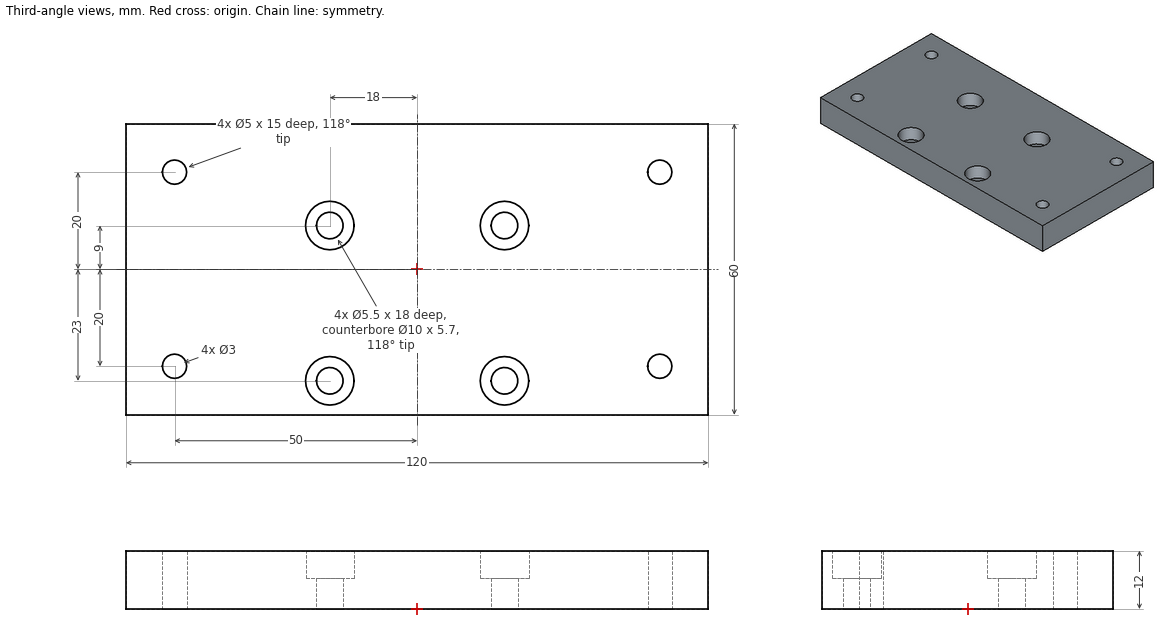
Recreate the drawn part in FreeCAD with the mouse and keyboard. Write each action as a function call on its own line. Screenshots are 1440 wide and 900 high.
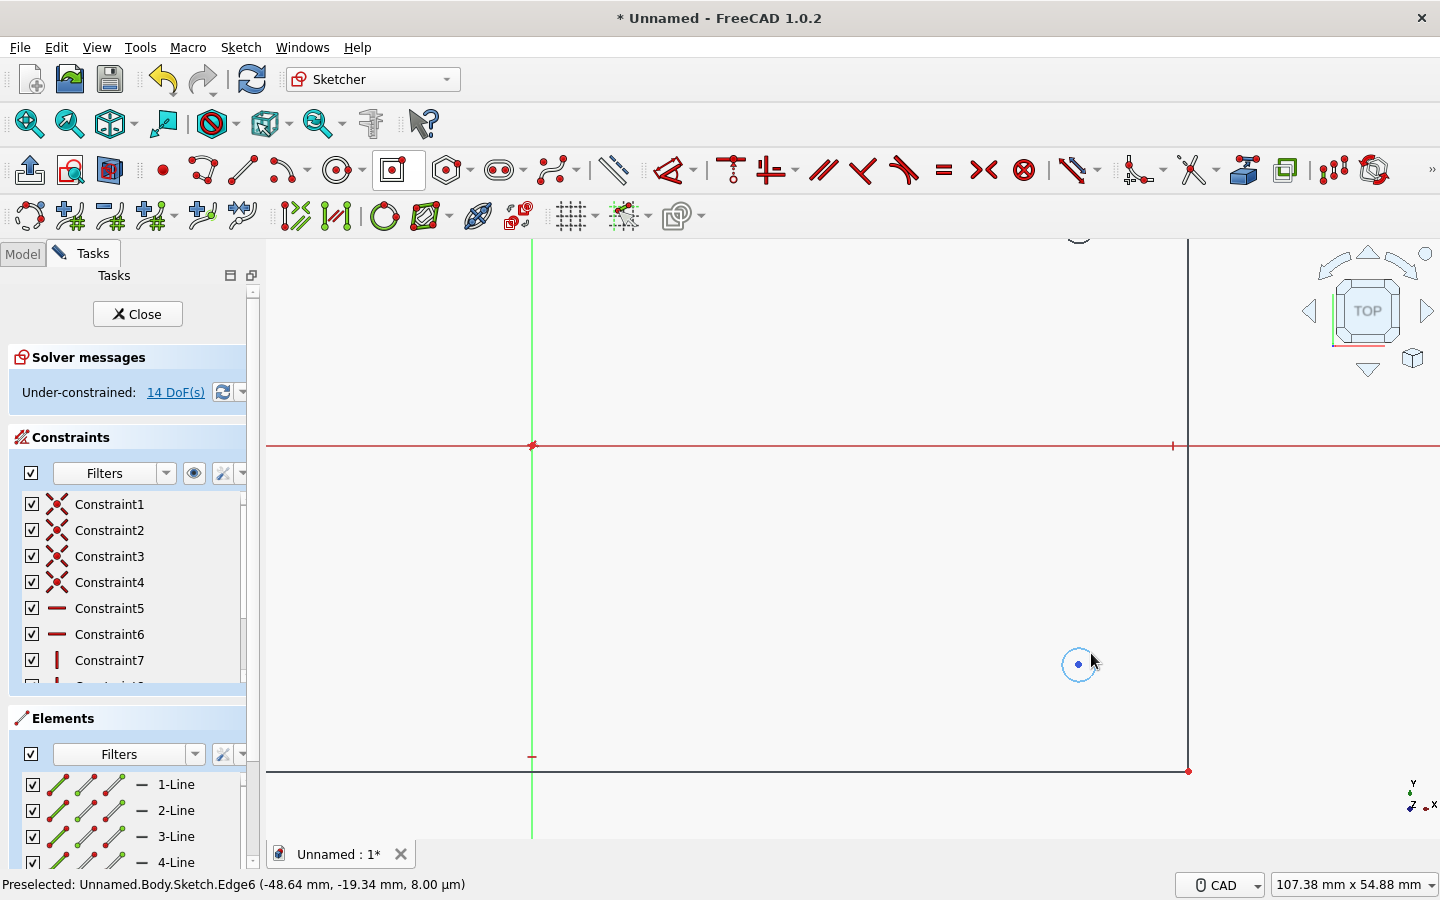
click(1091, 653)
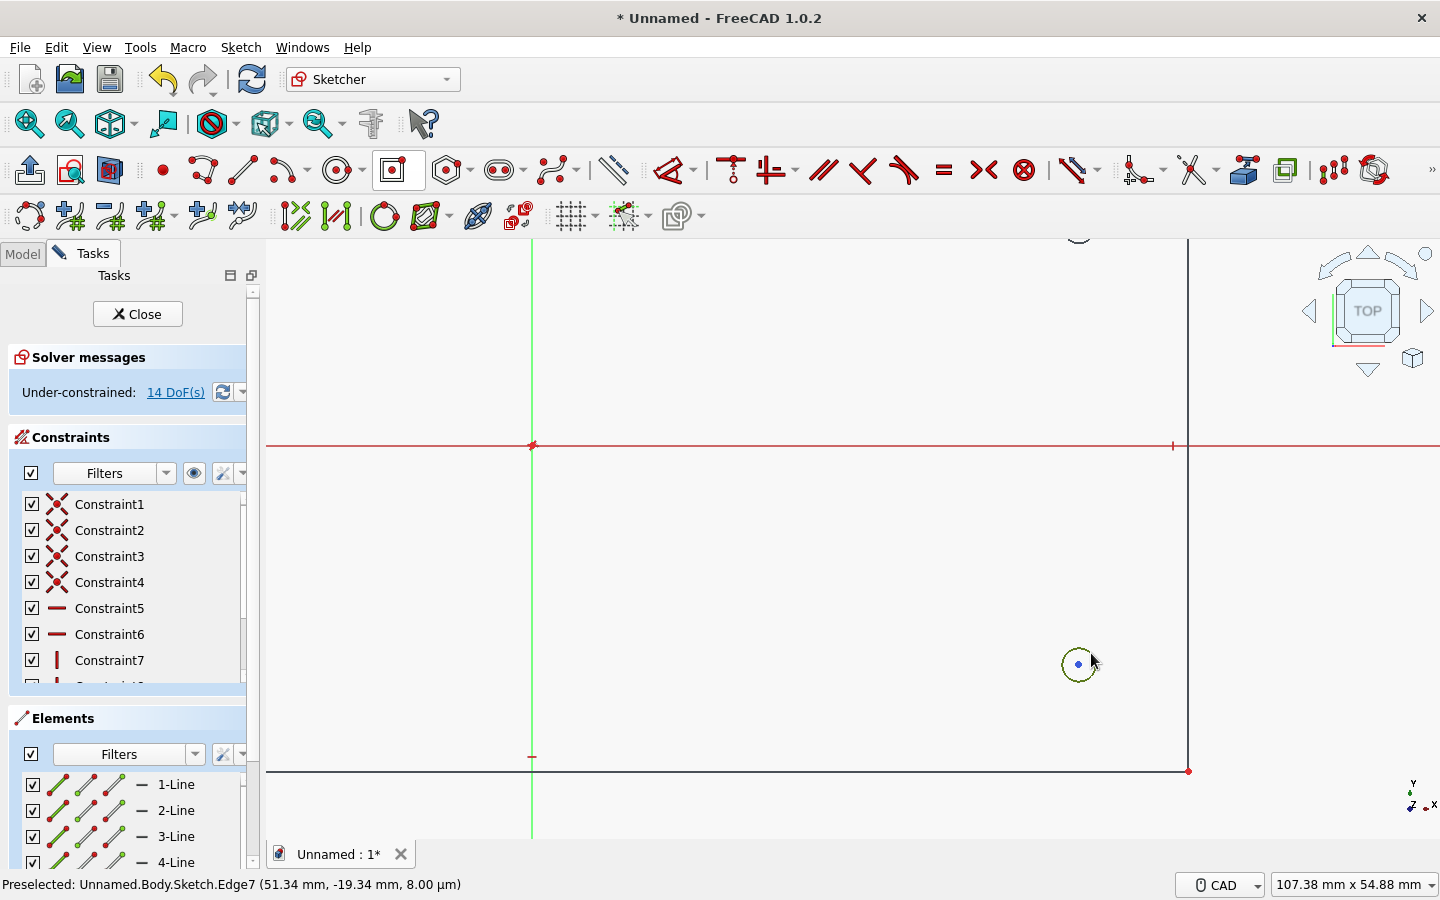
scroll(1091, 653, down, 3)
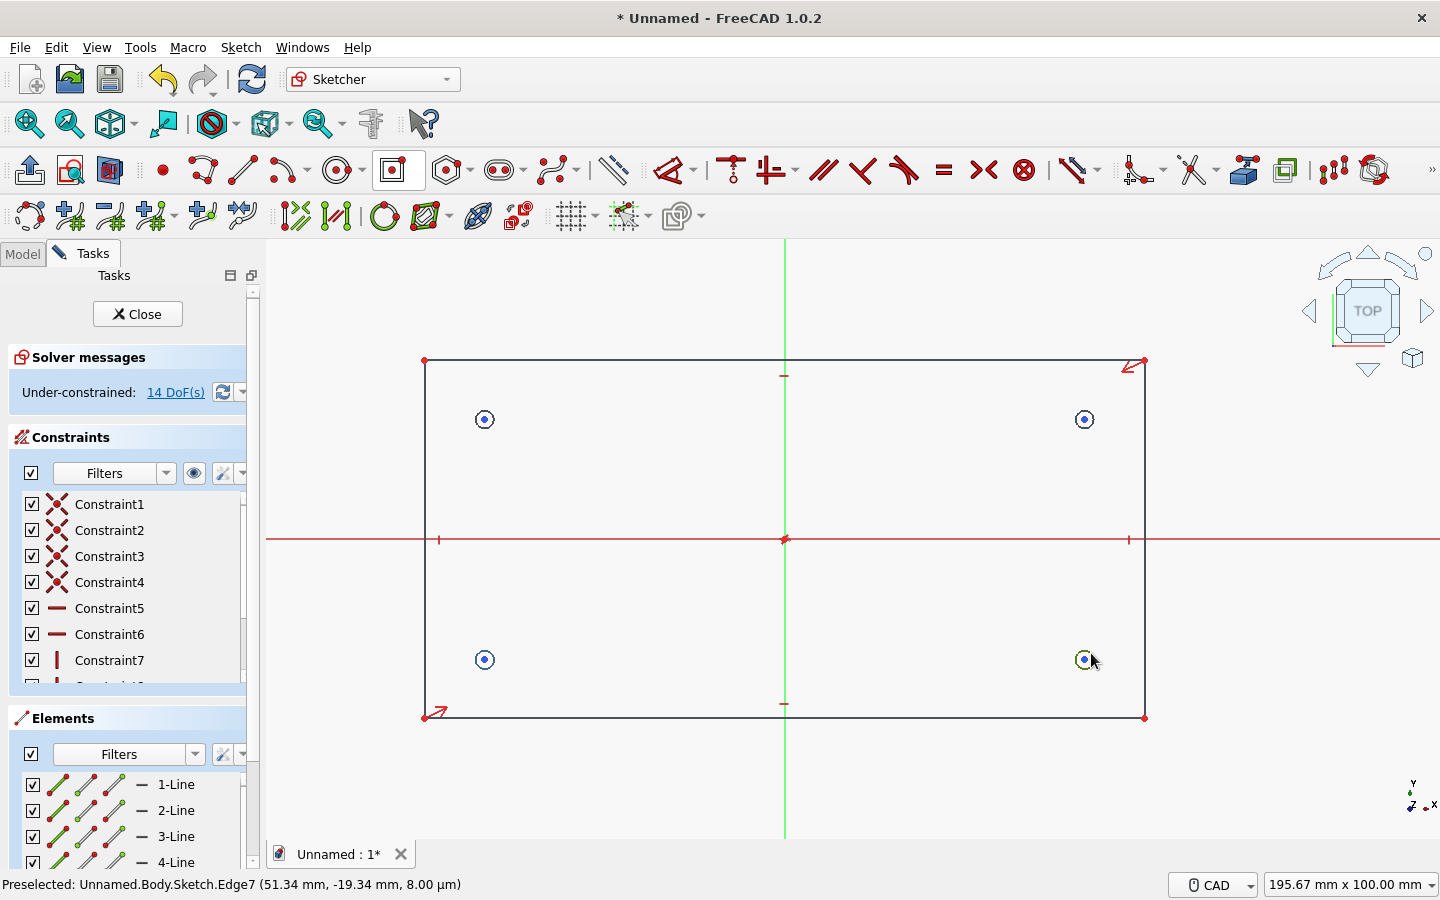
scroll(491, 413, up, 3)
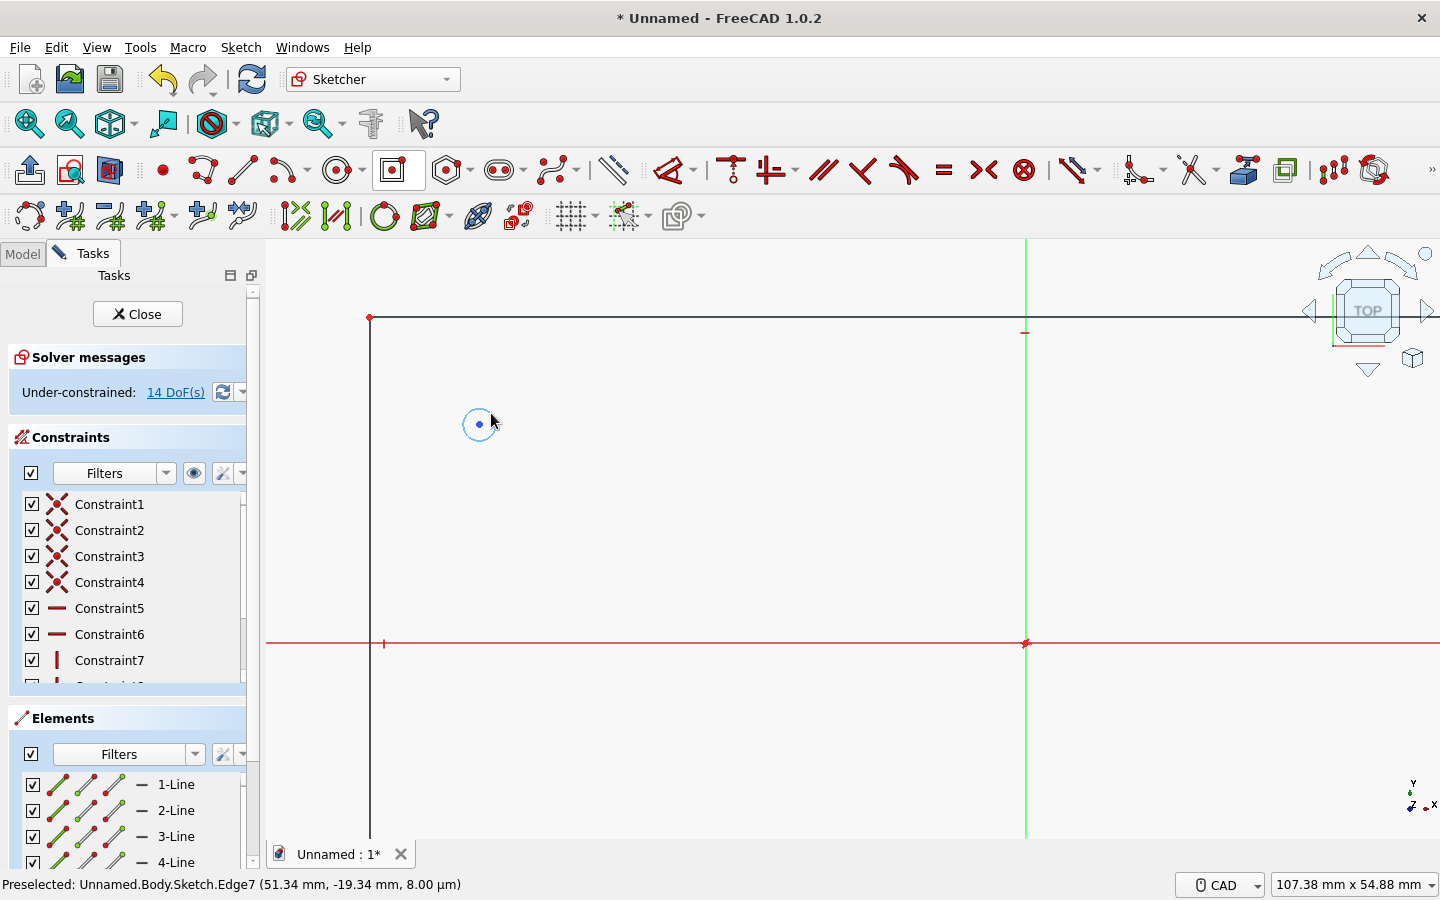
click(491, 413)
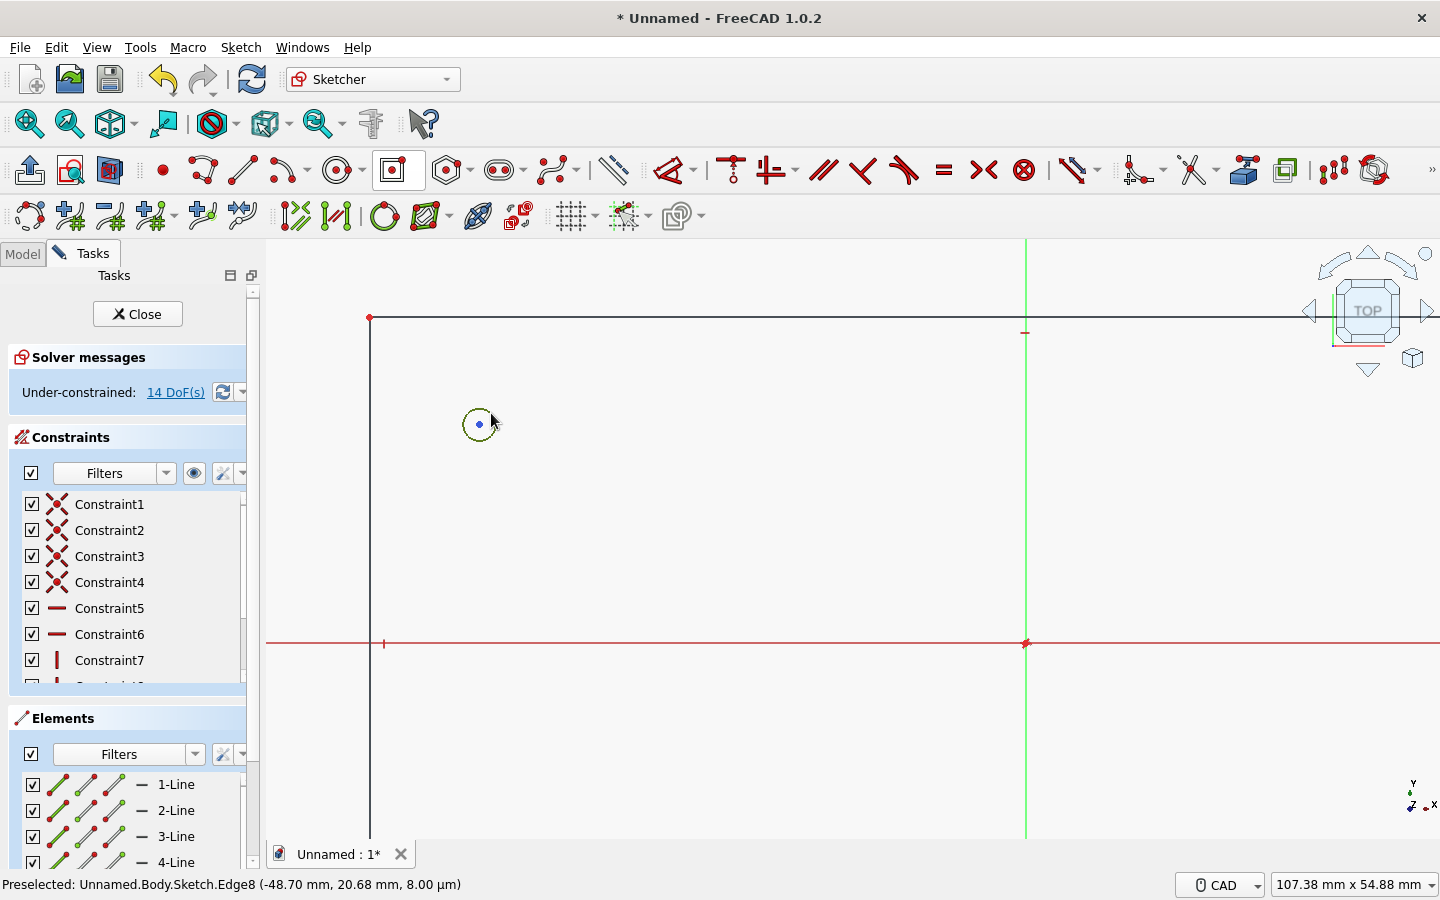
scroll(491, 412, down, 3)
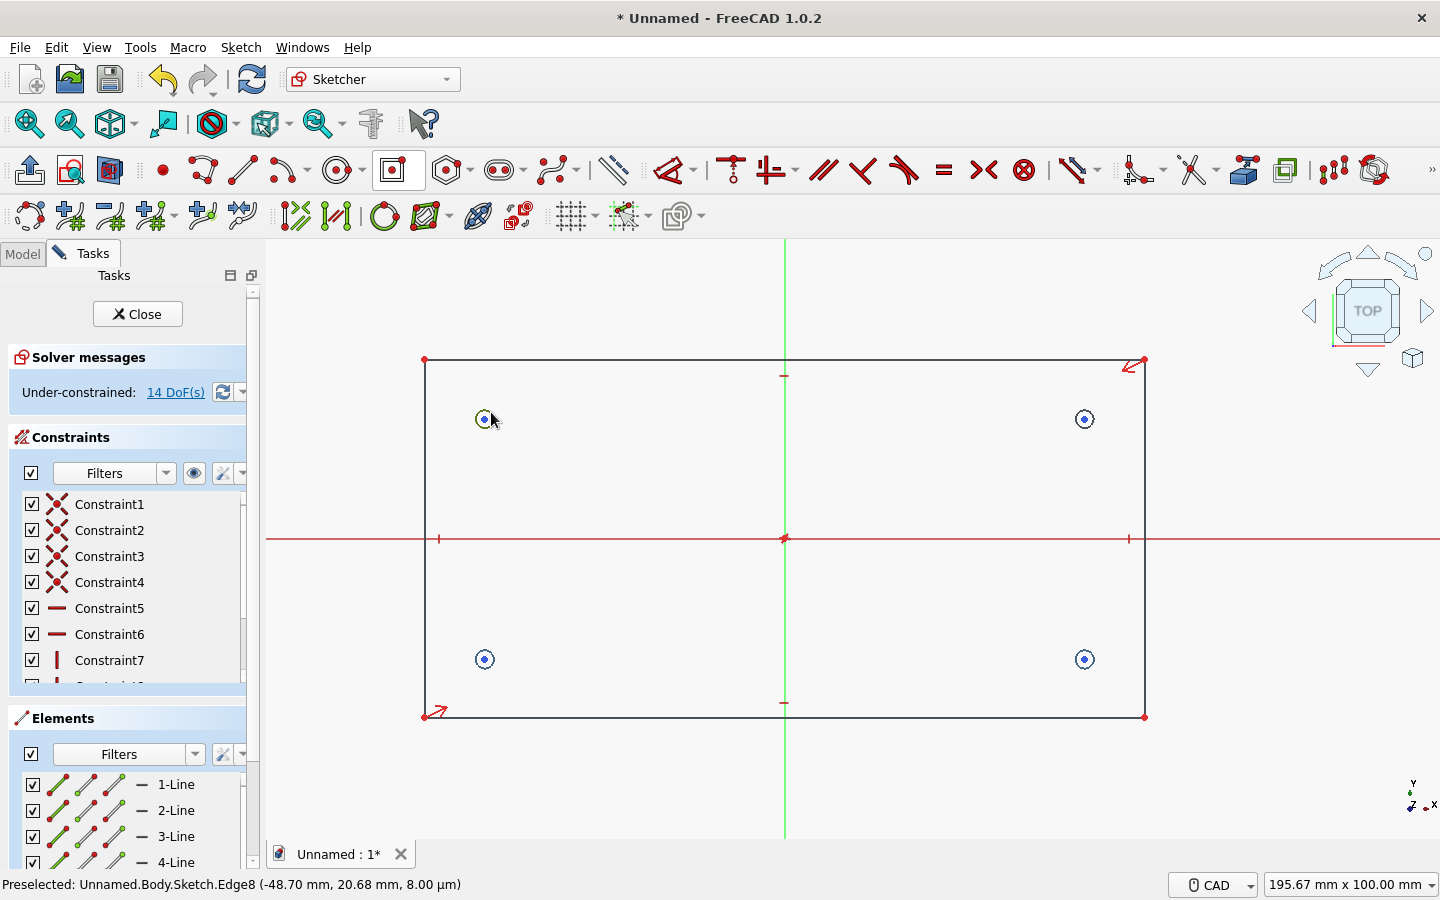
scroll(1091, 413, up, 3)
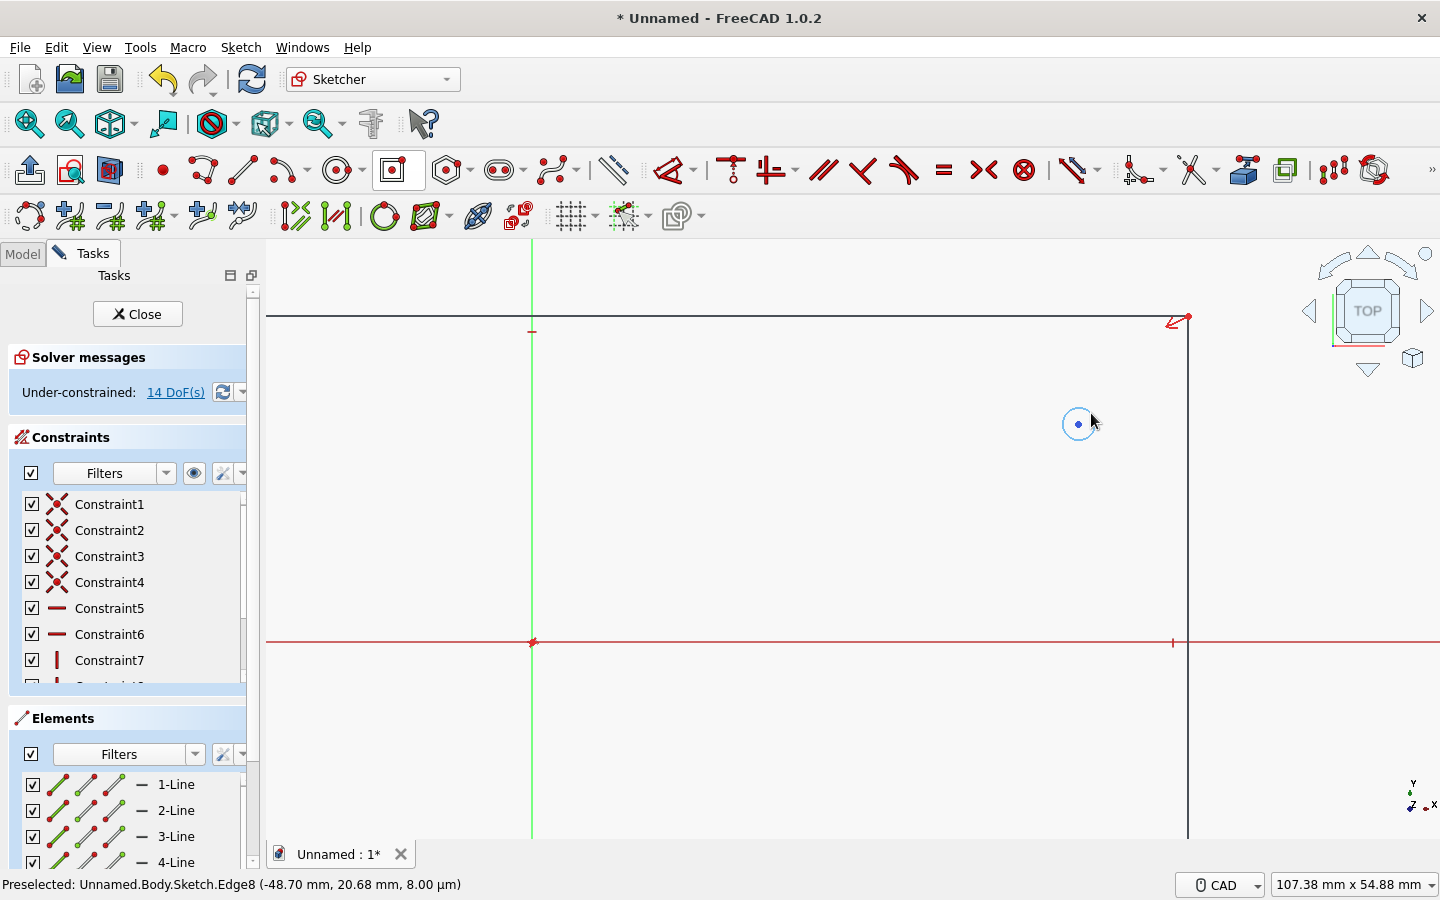
click(1090, 413)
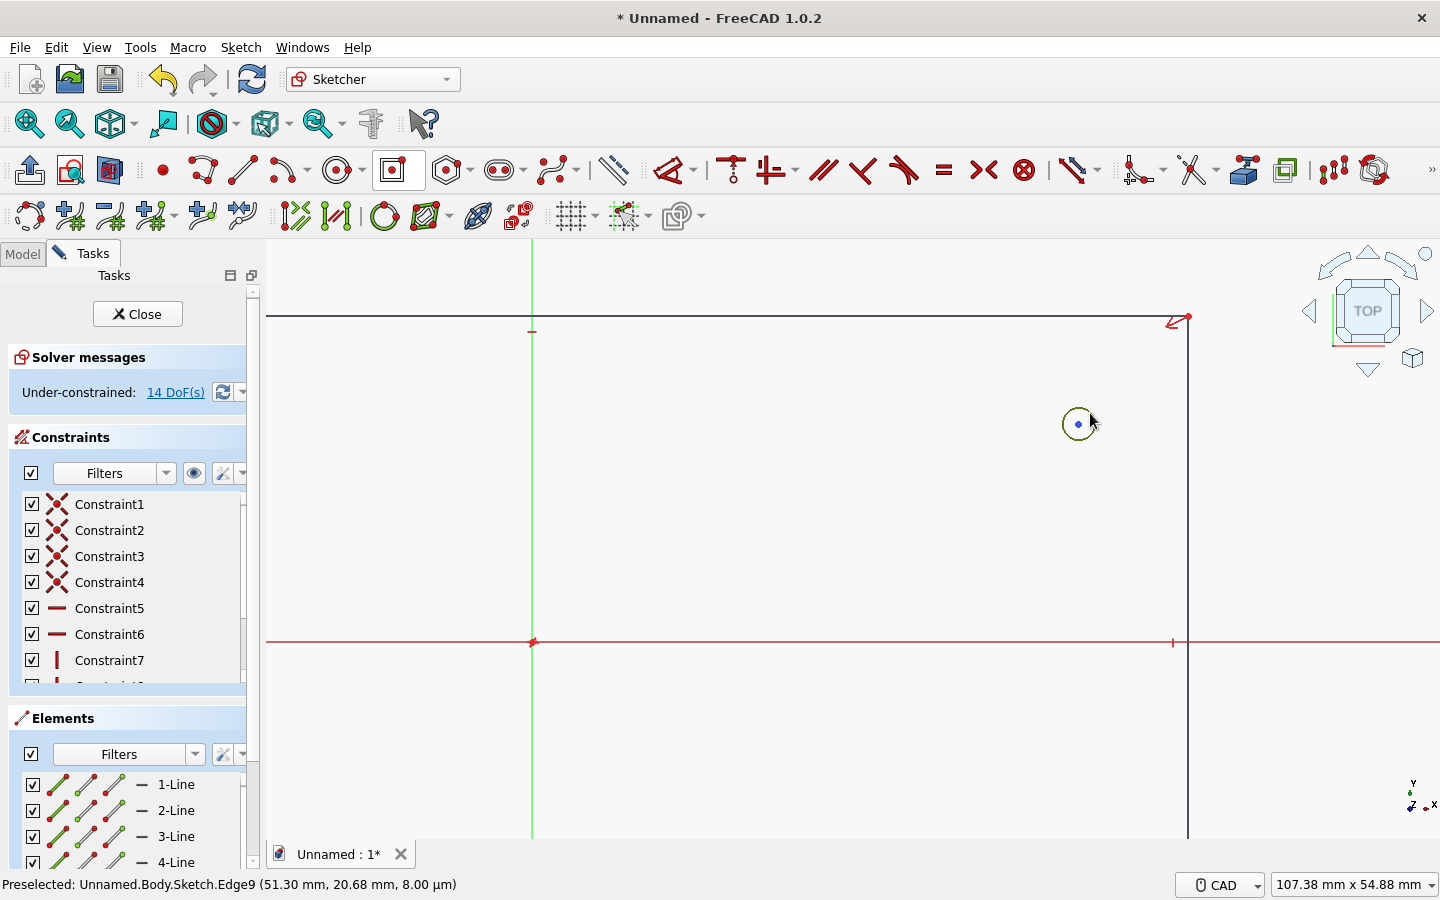
click(944, 170)